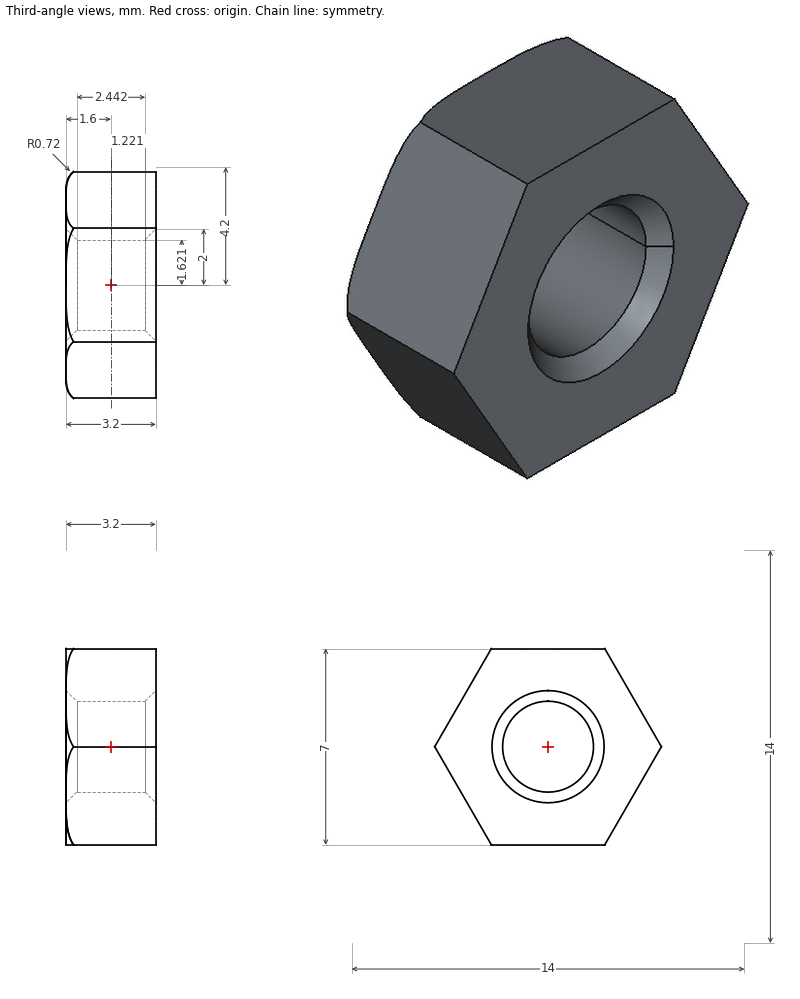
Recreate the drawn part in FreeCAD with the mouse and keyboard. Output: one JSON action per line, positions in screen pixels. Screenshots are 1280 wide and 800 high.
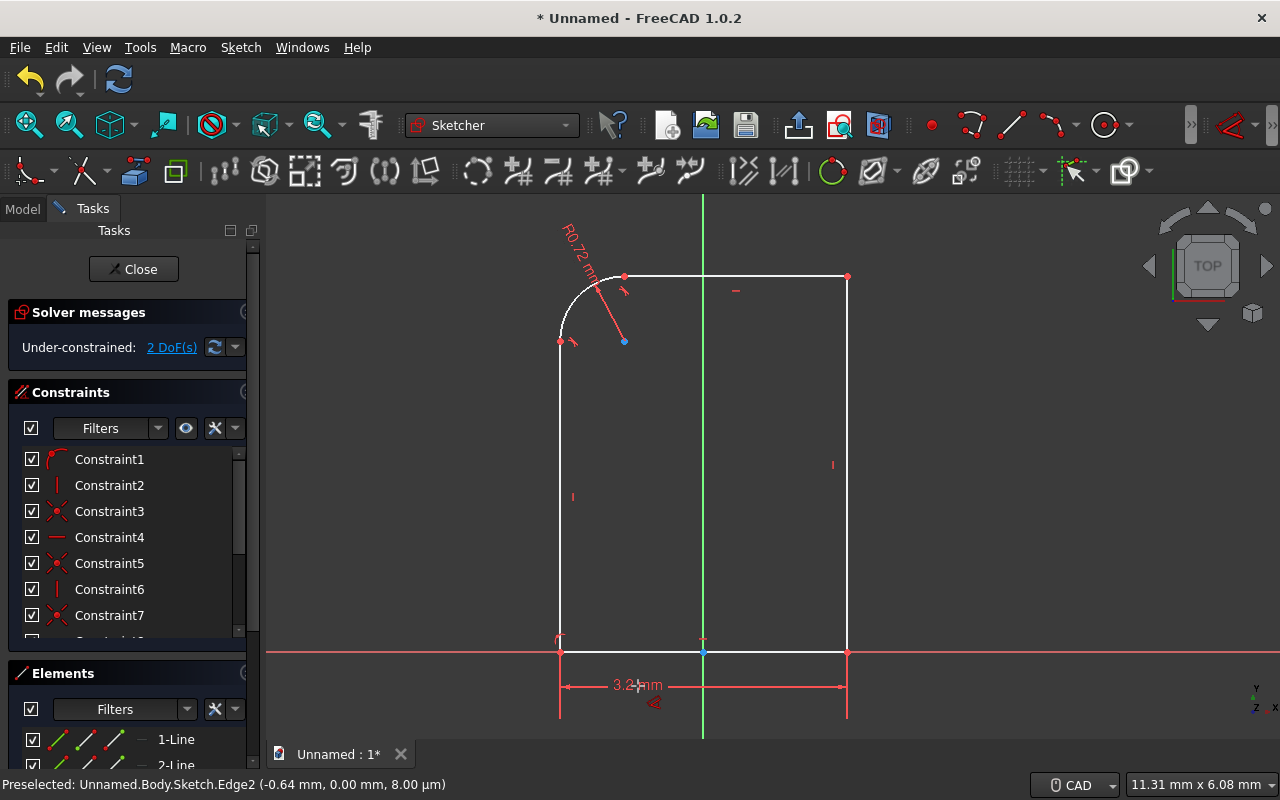
{"action": "left_click", "coordinate": [847, 539]}
{"action": "left_click", "coordinate": [881, 464]}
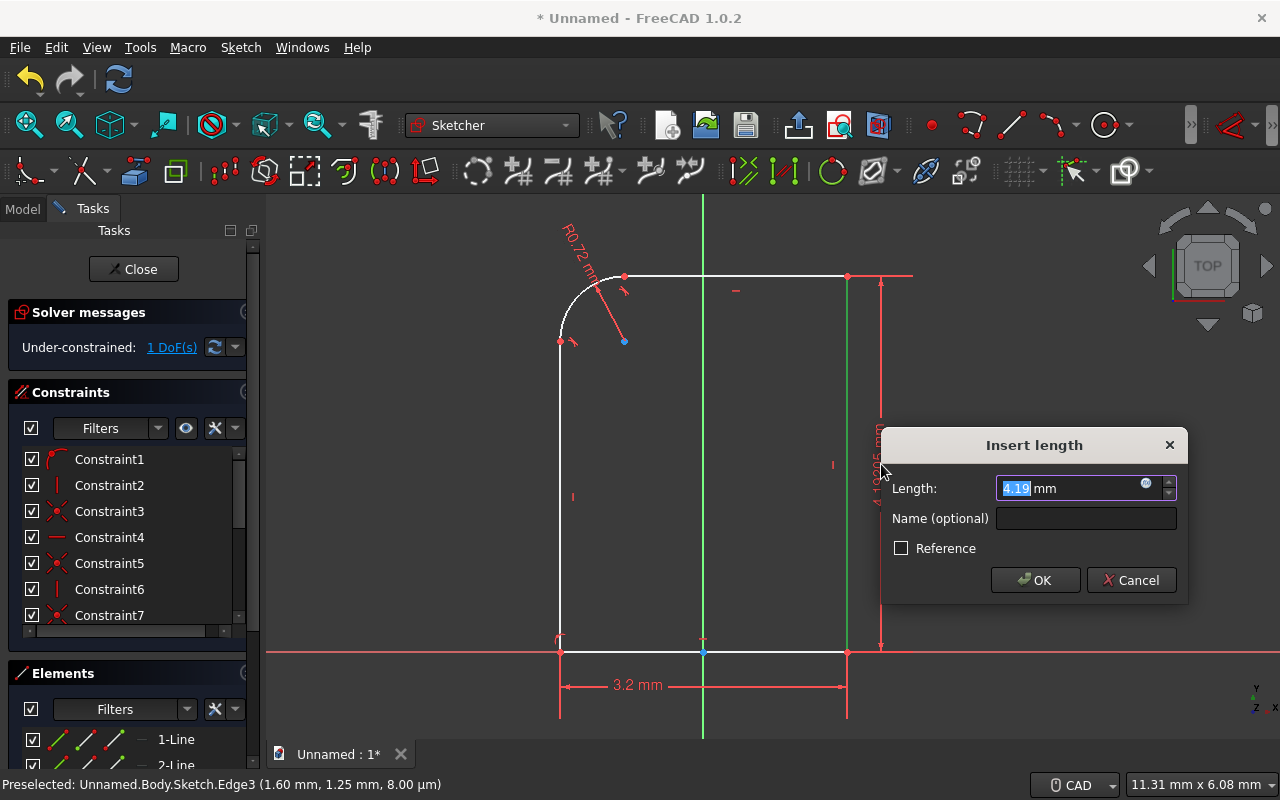
{"action": "type", "text": "4.2"}
{"action": "key", "text": "Return"}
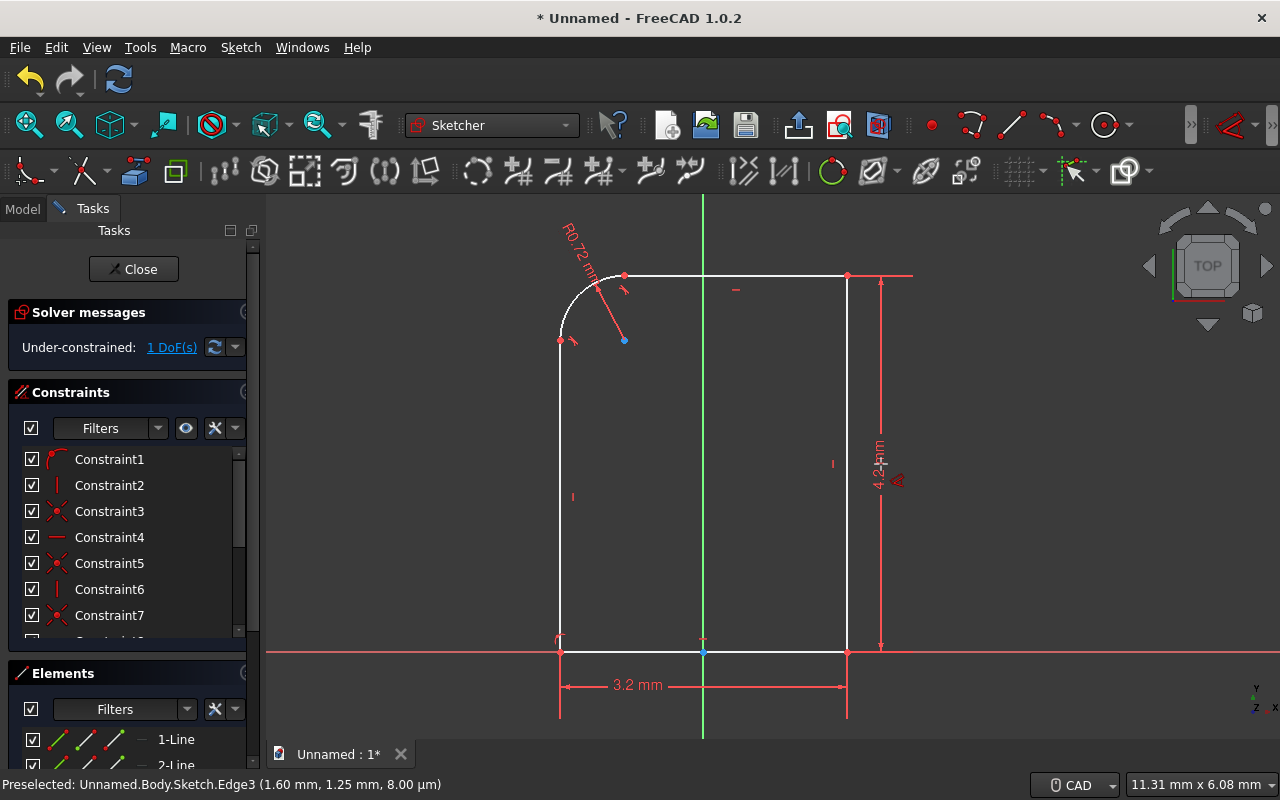
{"action": "left_click", "coordinate": [560, 340]}
{"action": "left_click", "coordinate": [632, 306]}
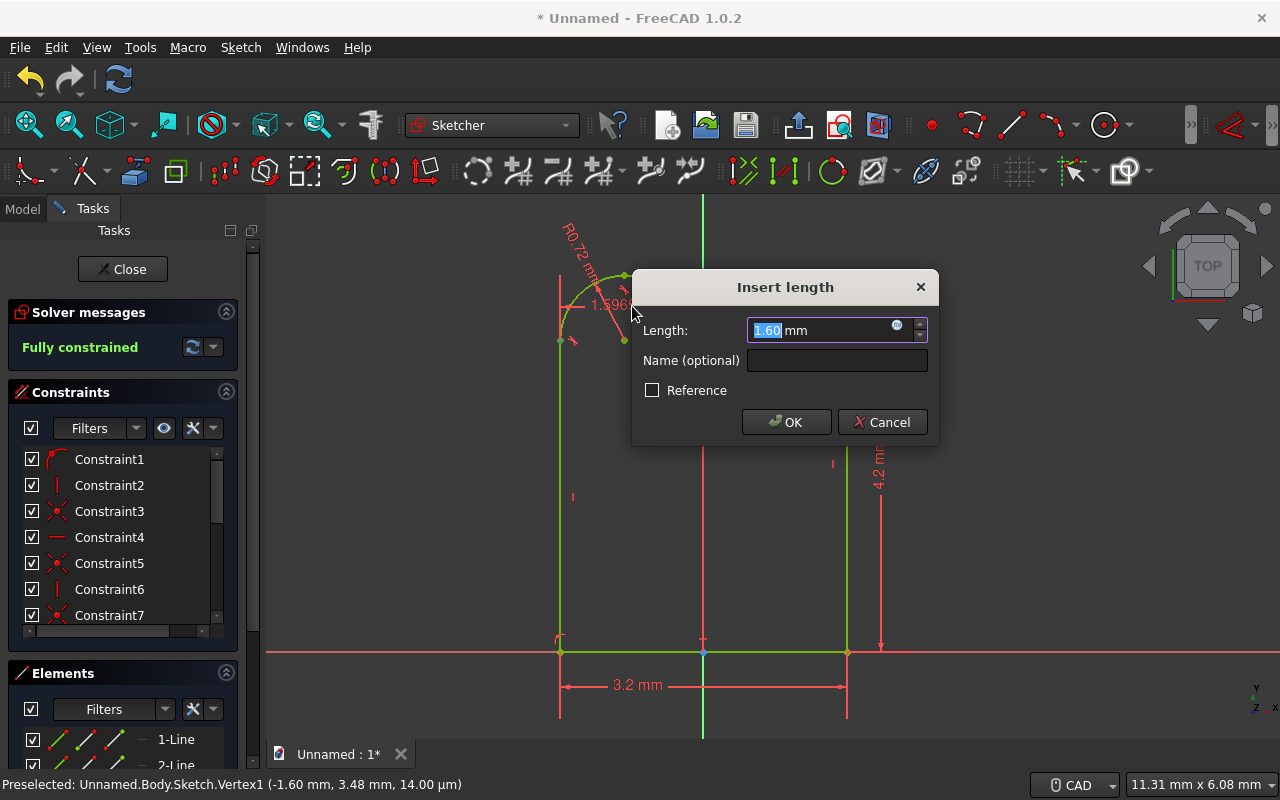
{"action": "type", "text": "1.6"}
{"action": "key", "text": "Return"}
{"action": "key", "text": "Escape"}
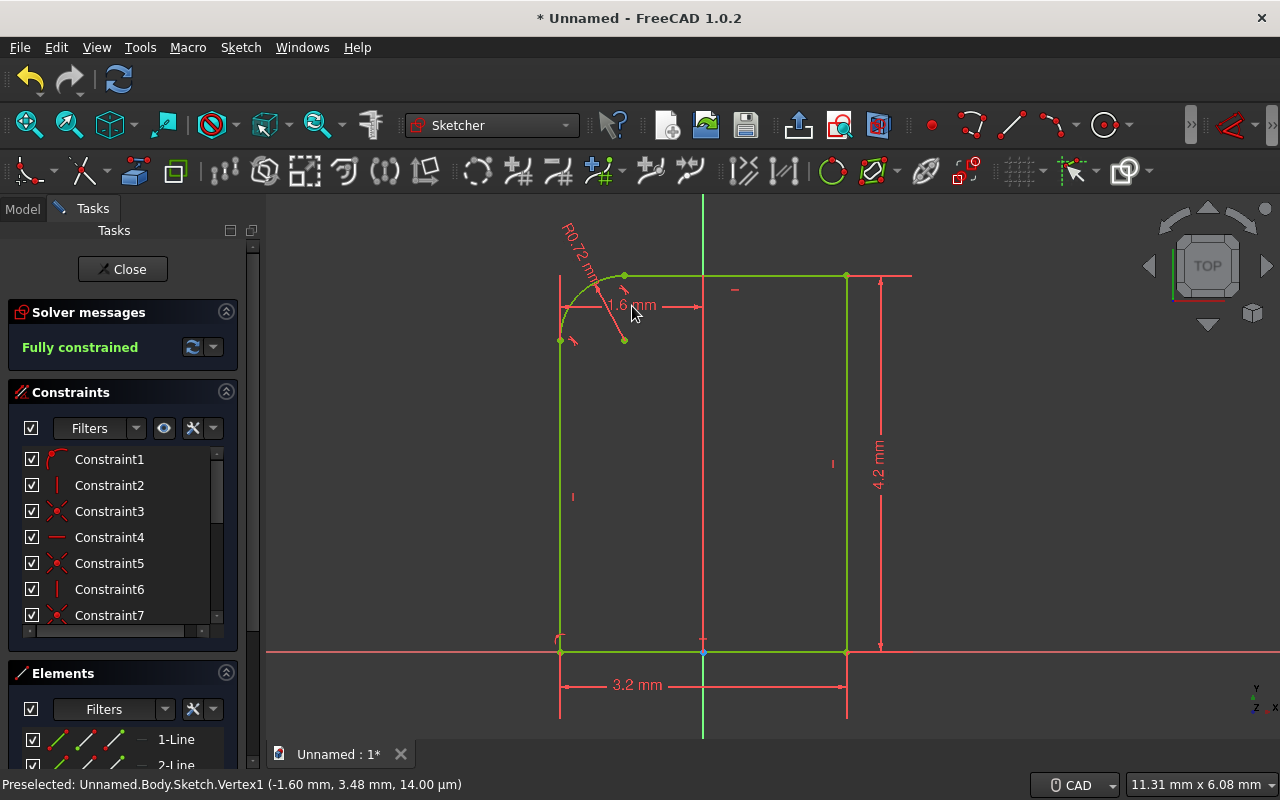
{"action": "left_click", "coordinate": [123, 269]}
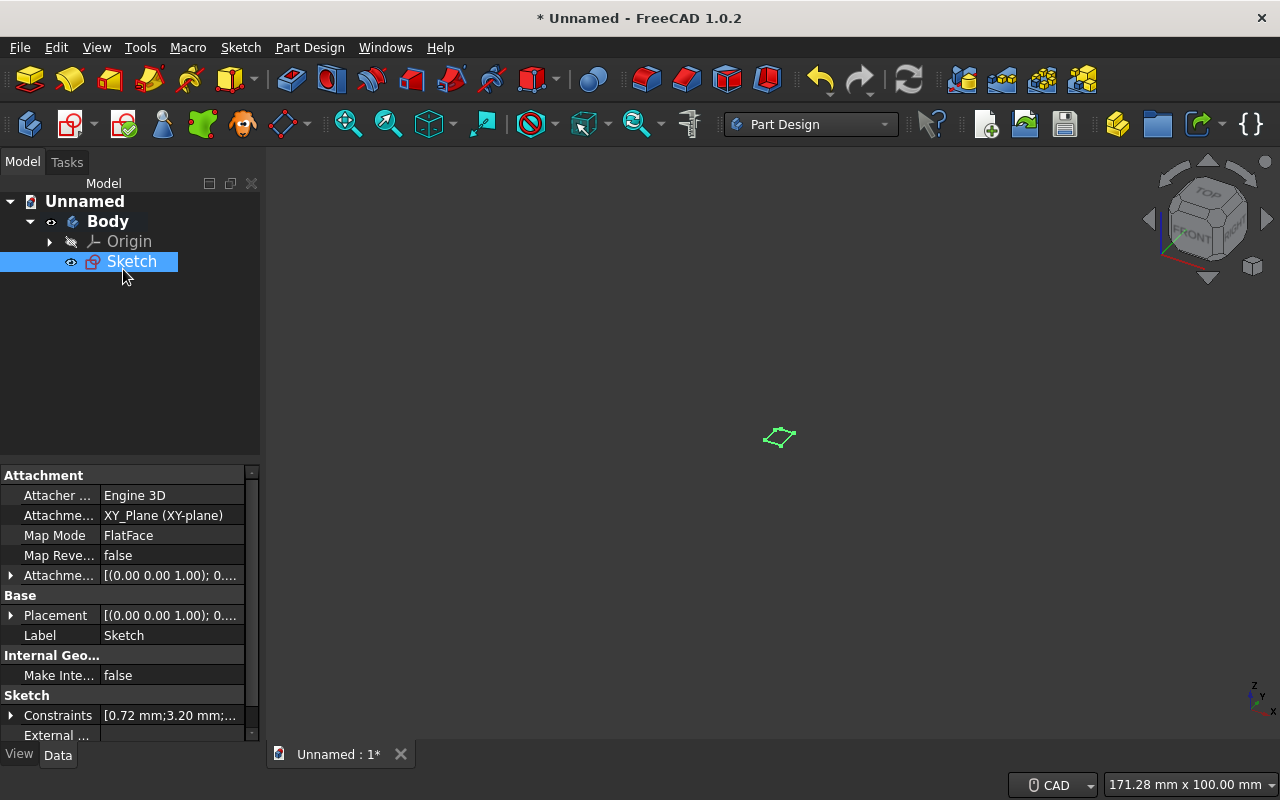
{"action": "left_click", "coordinate": [70, 80]}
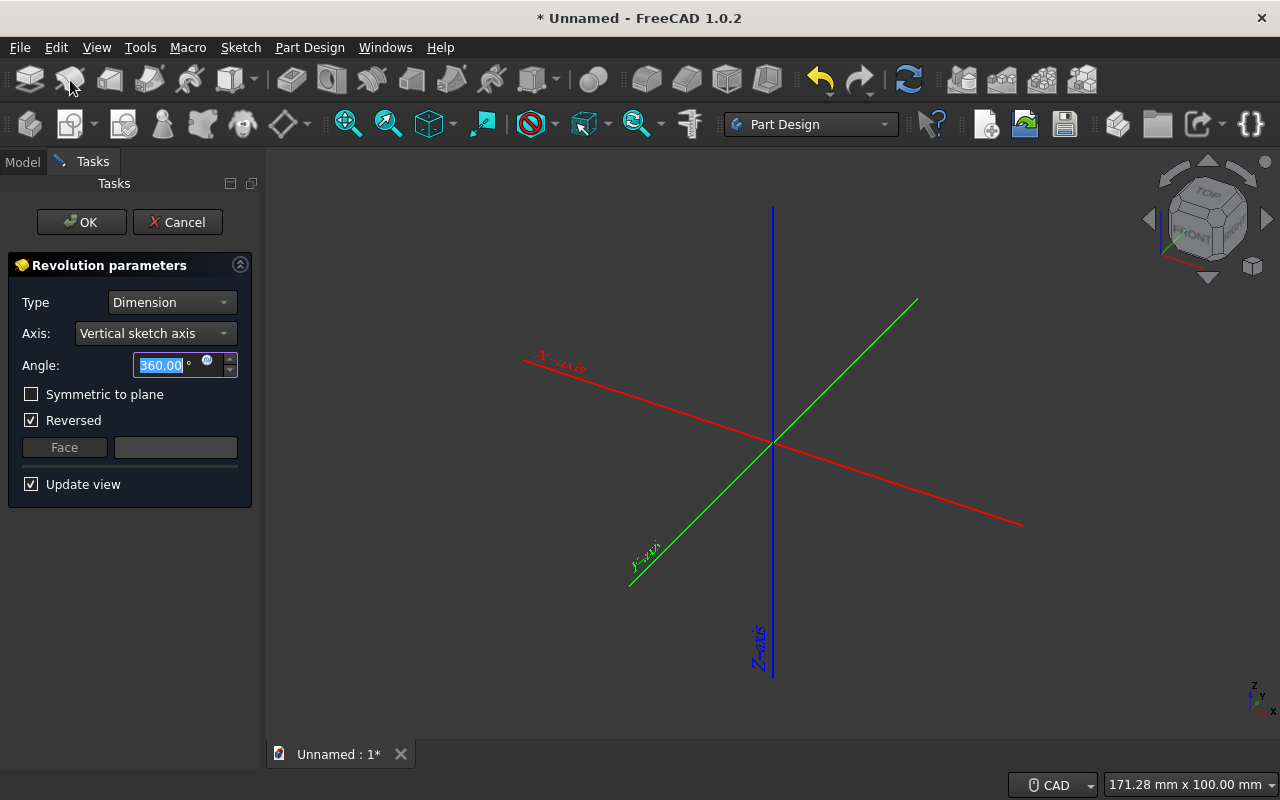
{"action": "left_click", "coordinate": [156, 334]}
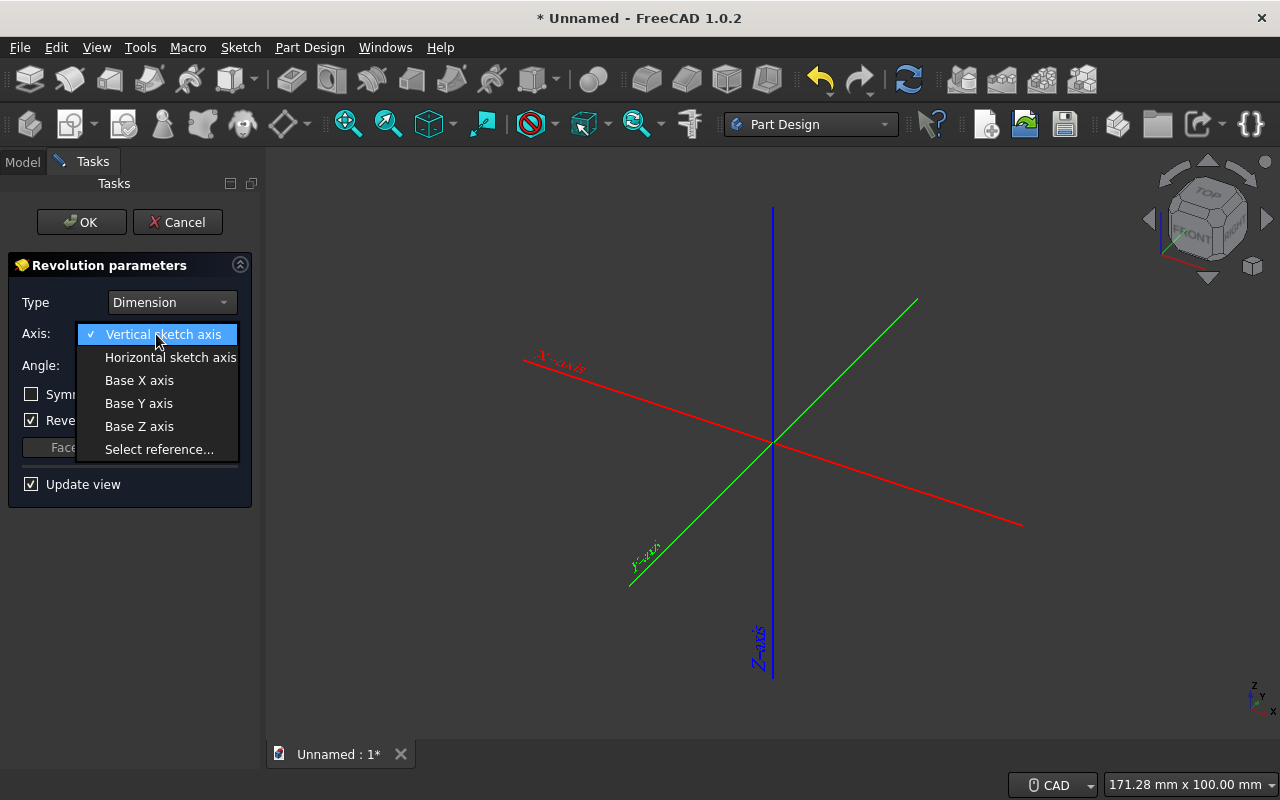
{"action": "left_click", "coordinate": [156, 358]}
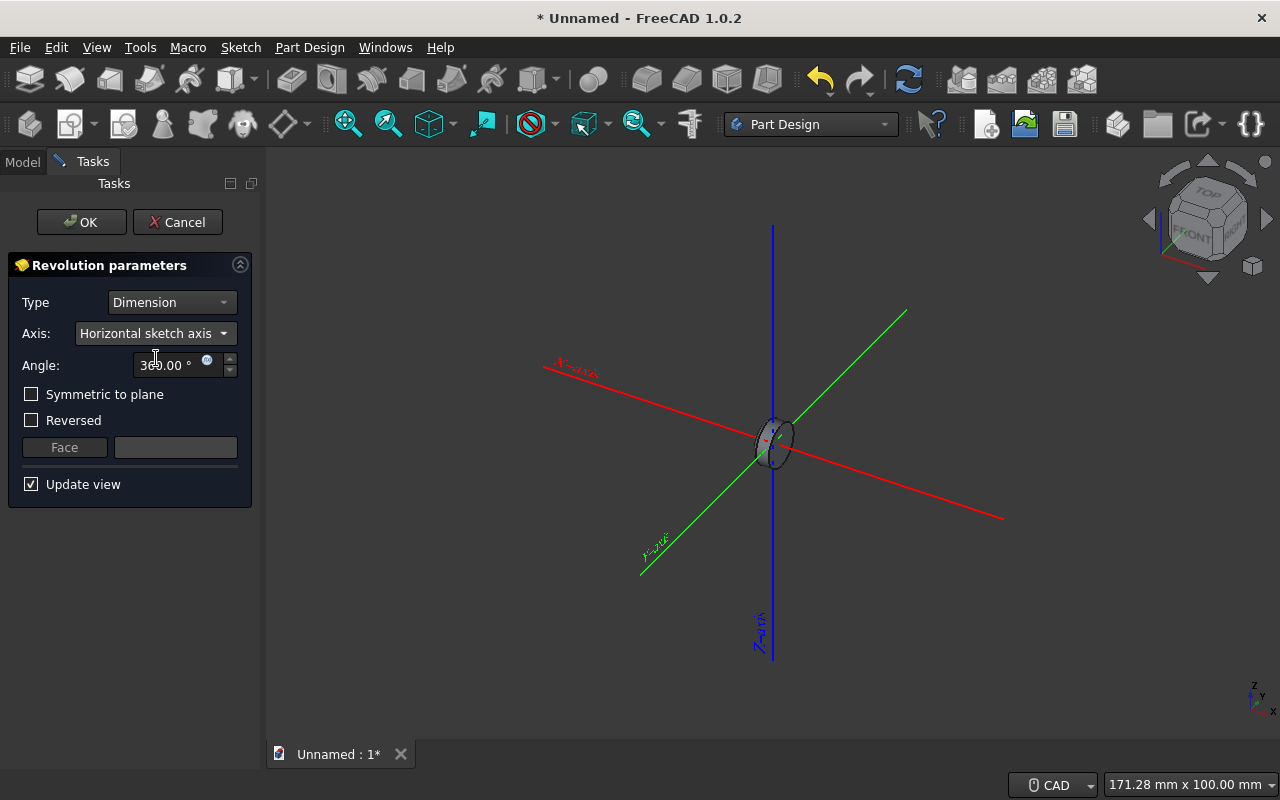
{"action": "left_click", "coordinate": [82, 222]}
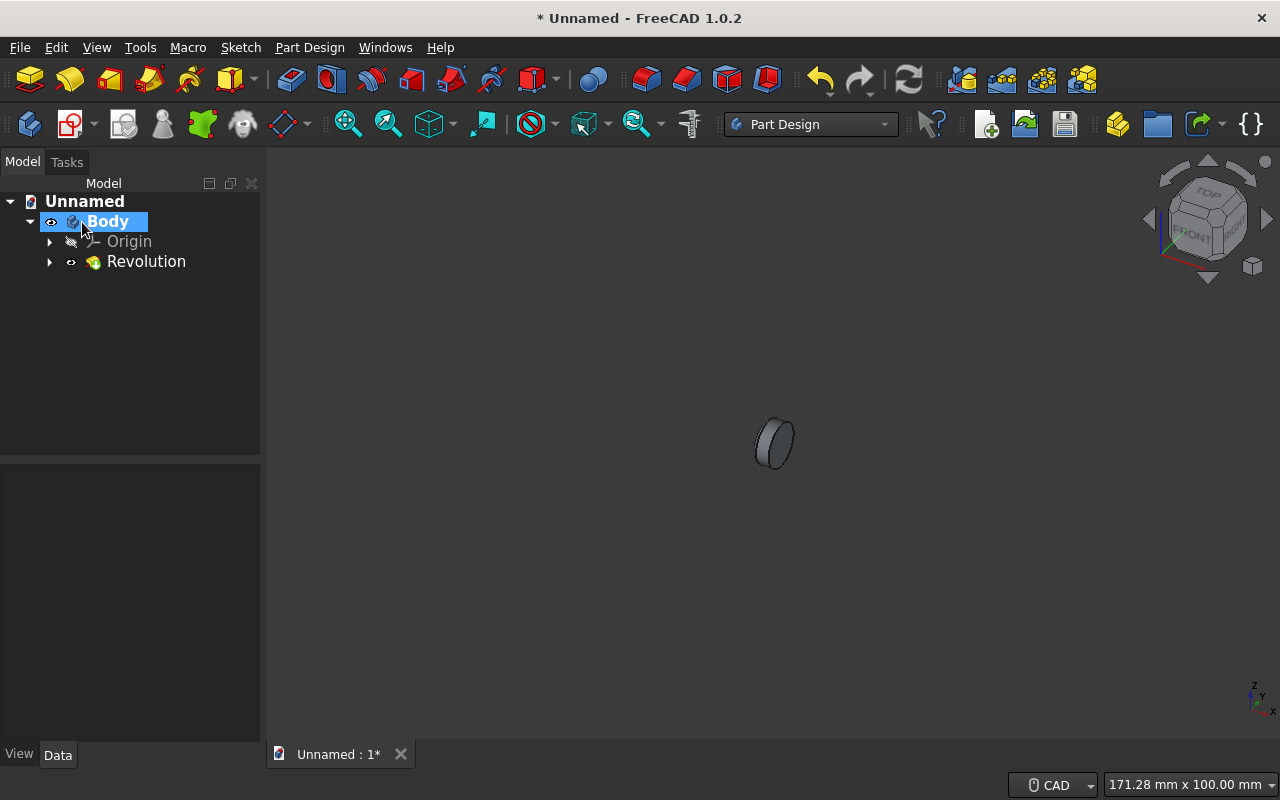
{"action": "key", "text": "v f"}